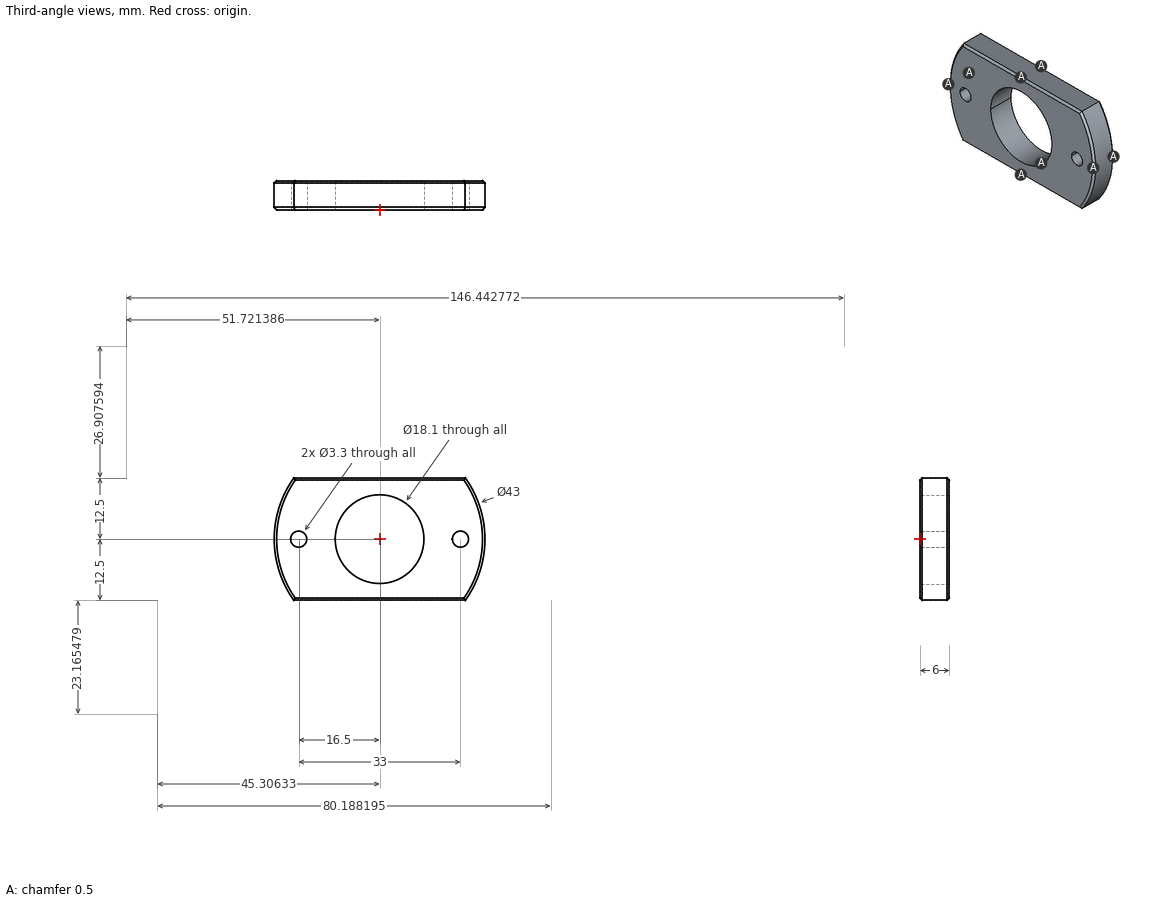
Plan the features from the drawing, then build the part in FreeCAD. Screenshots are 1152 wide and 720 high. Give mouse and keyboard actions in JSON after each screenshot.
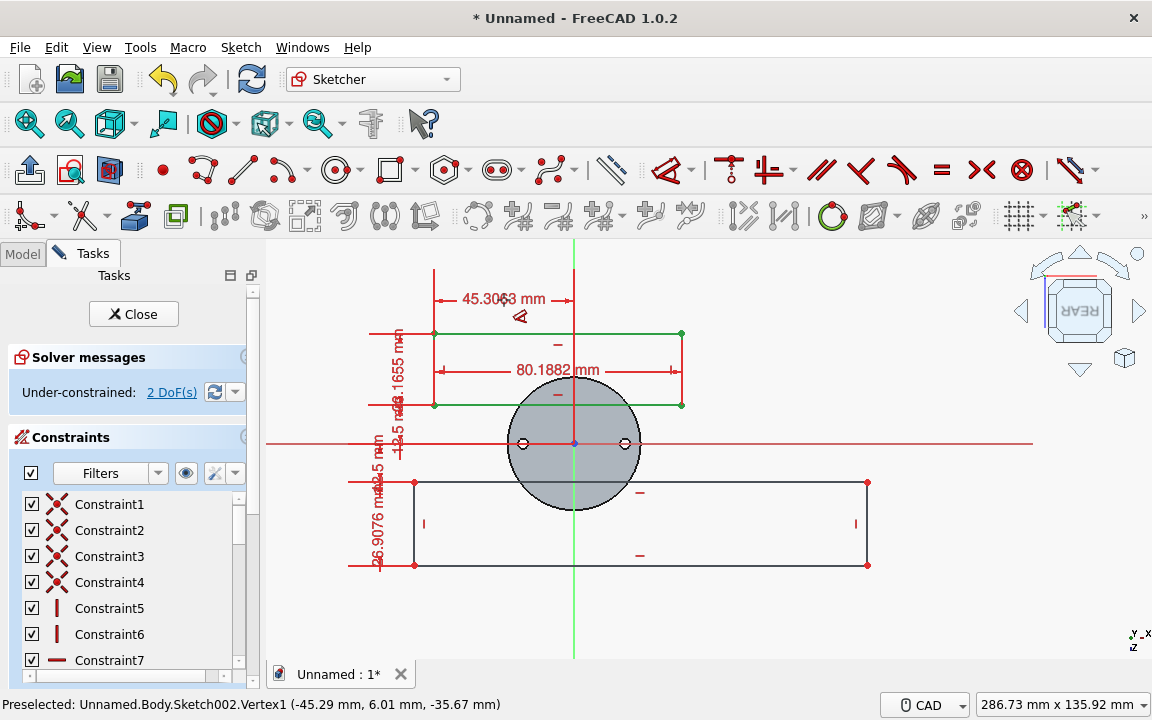
{"action": "left_click", "coordinate": [550, 566]}
{"action": "left_click", "coordinate": [641, 600]}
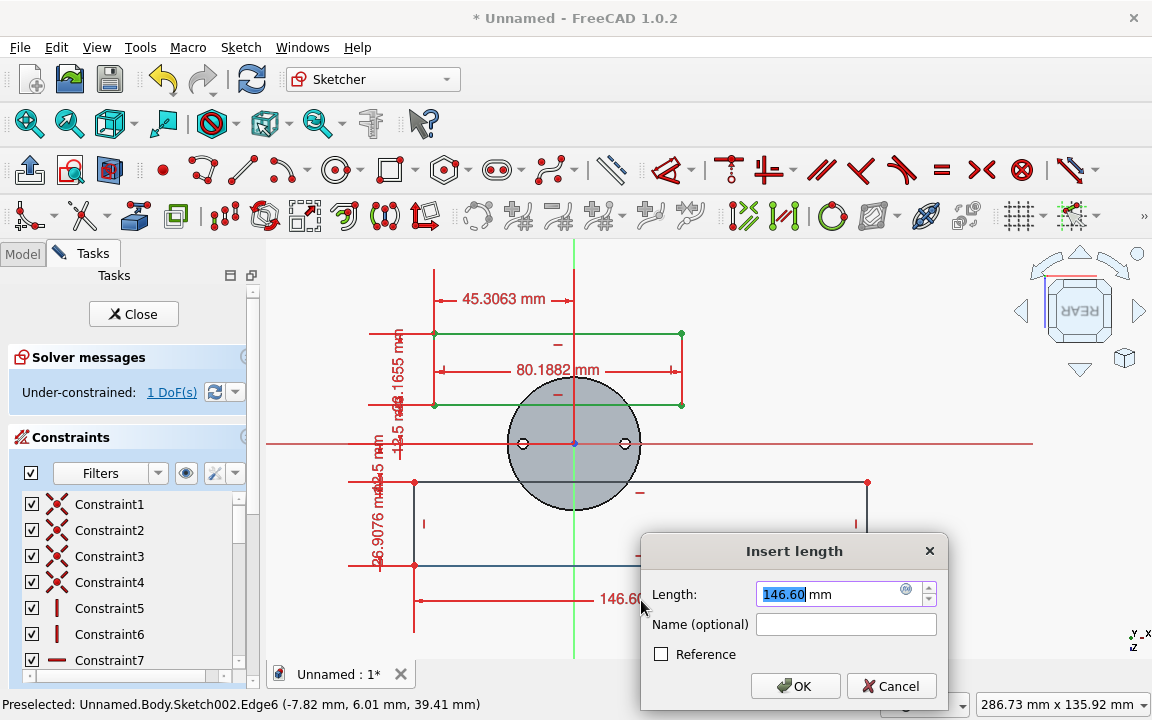
{"action": "type", "text": "146.442772"}
{"action": "key", "text": "Return"}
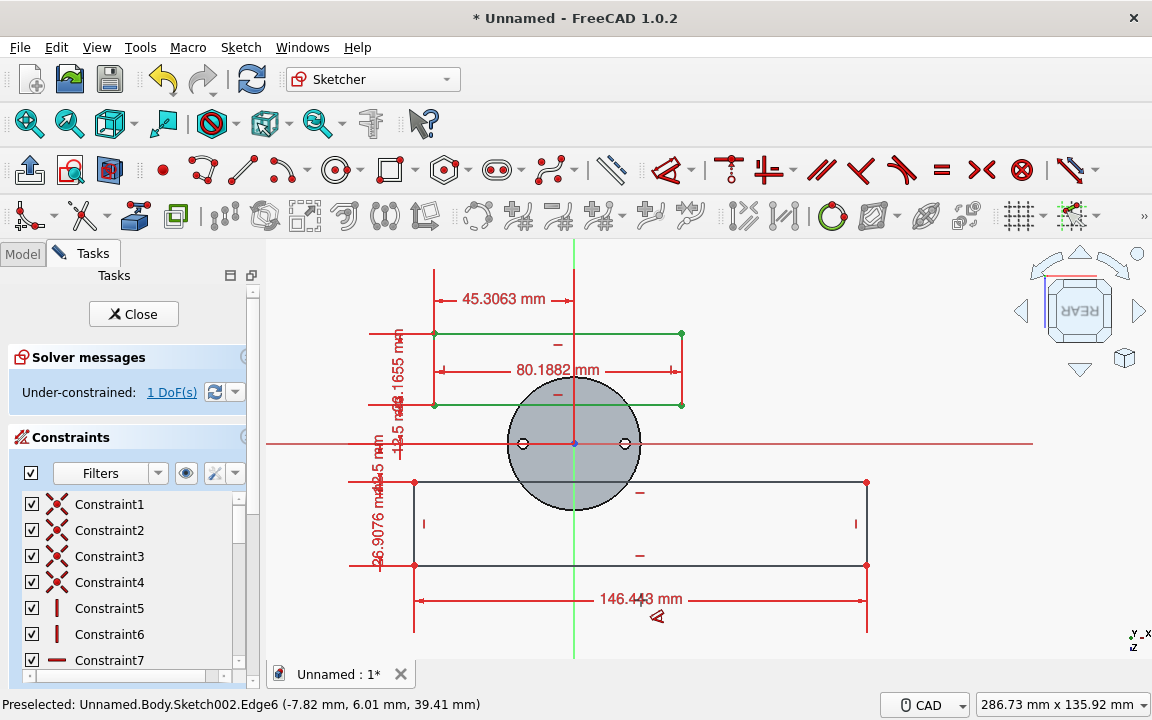
{"action": "left_click", "coordinate": [414, 482]}
{"action": "left_click", "coordinate": [494, 516]}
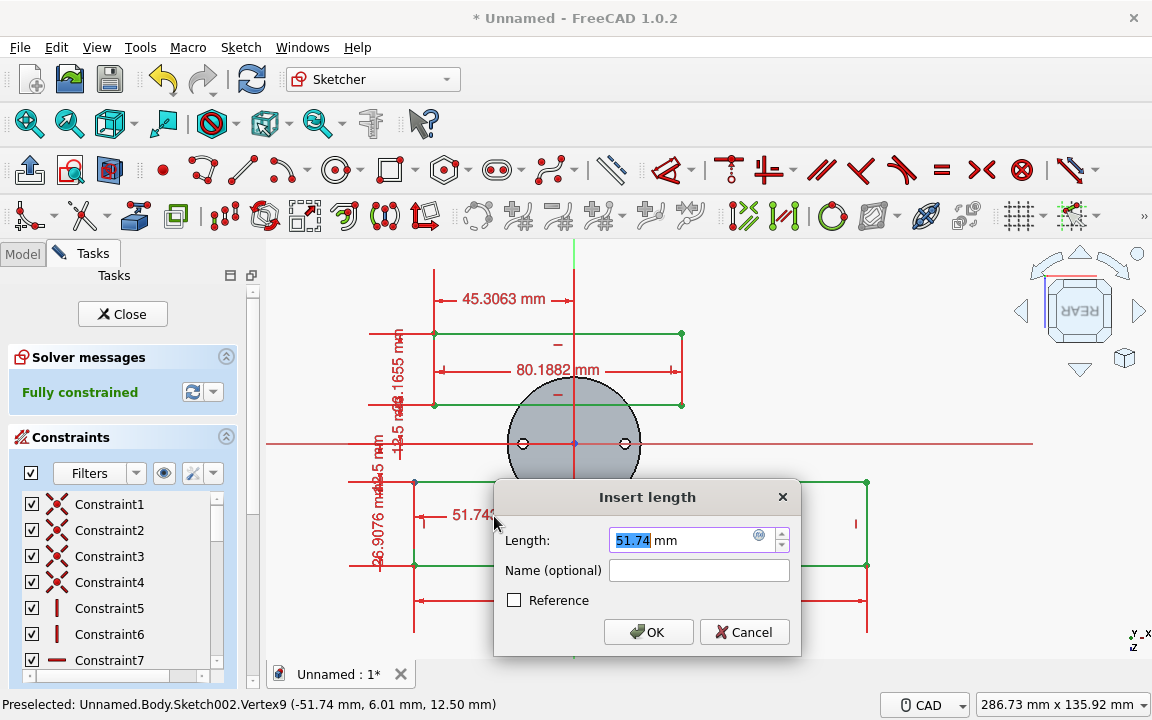
{"action": "type", "text": "51.721386"}
{"action": "key", "text": "Return"}
{"action": "key", "text": "Escape"}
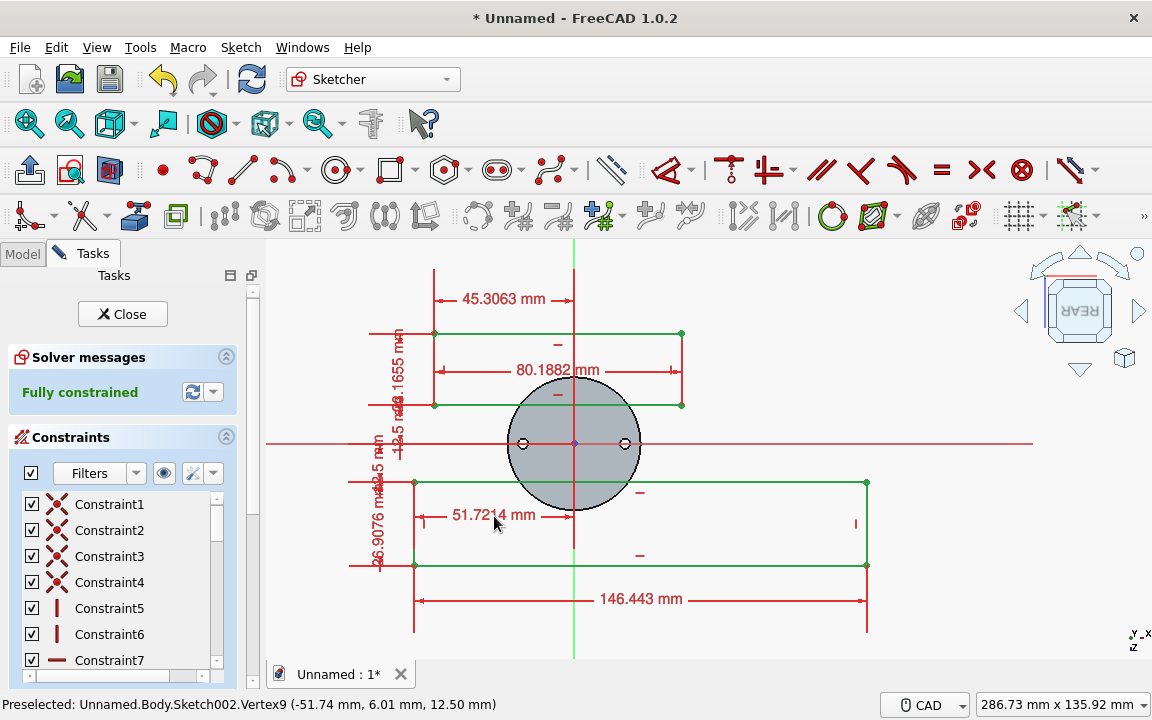
{"action": "left_click", "coordinate": [123, 314]}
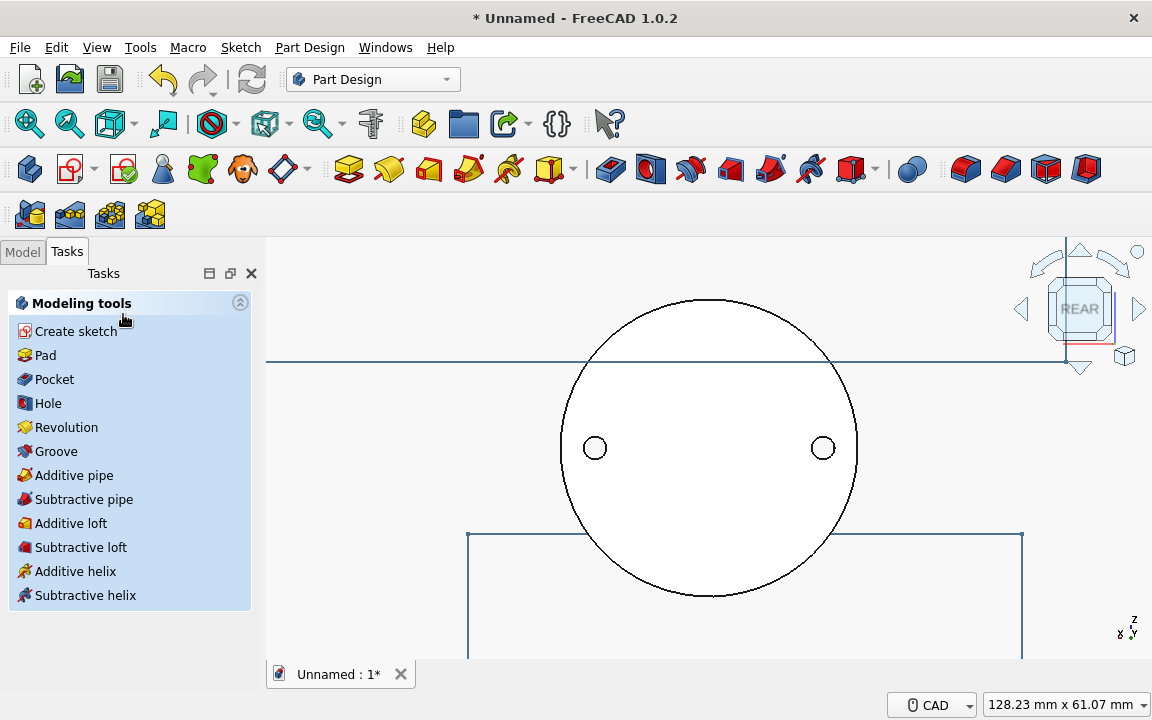
{"action": "left_click", "coordinate": [612, 170]}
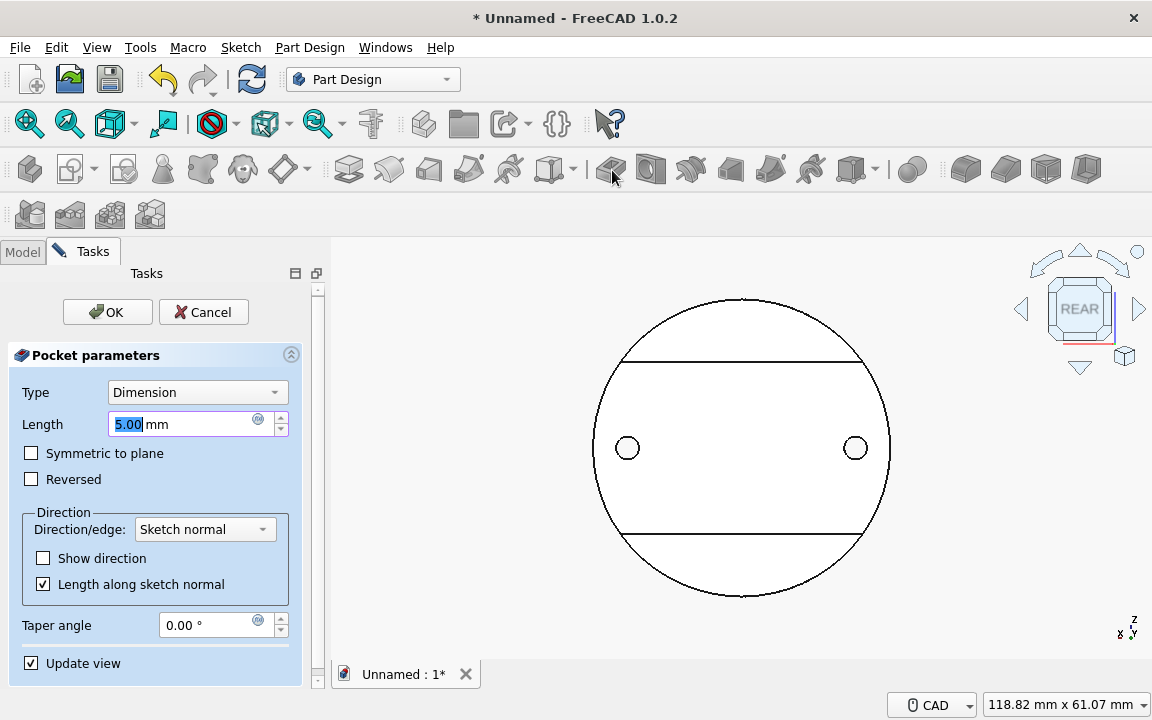
{"action": "left_click", "coordinate": [198, 392]}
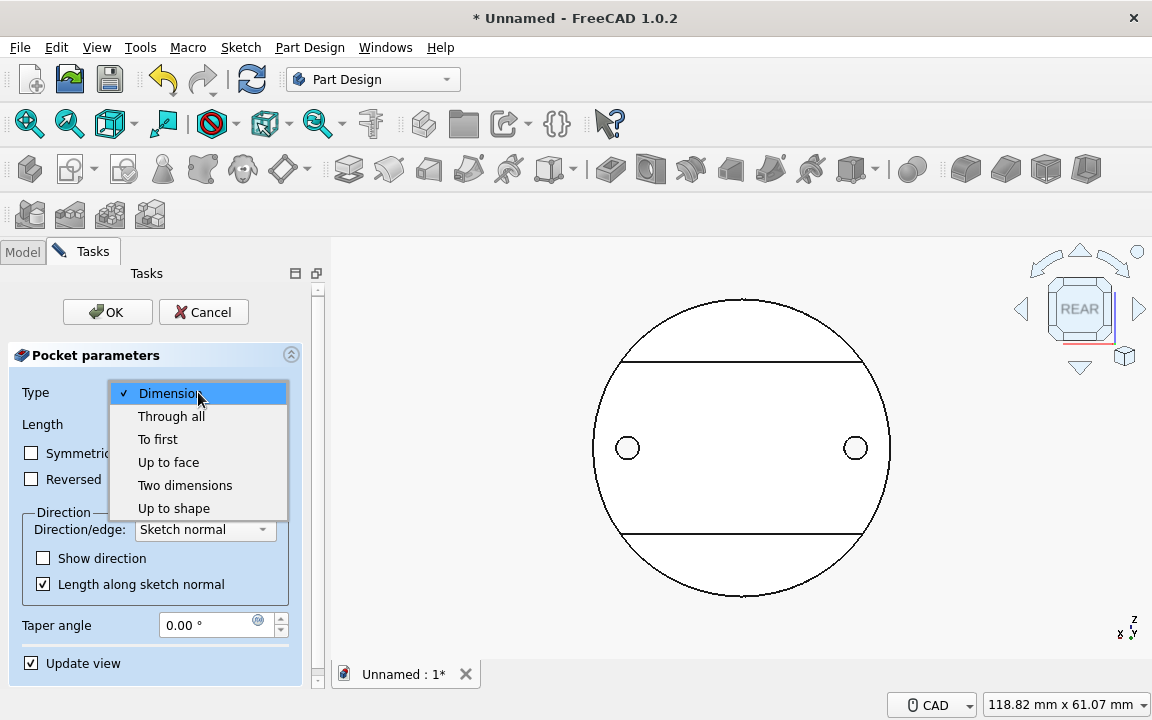
{"action": "left_click", "coordinate": [198, 416]}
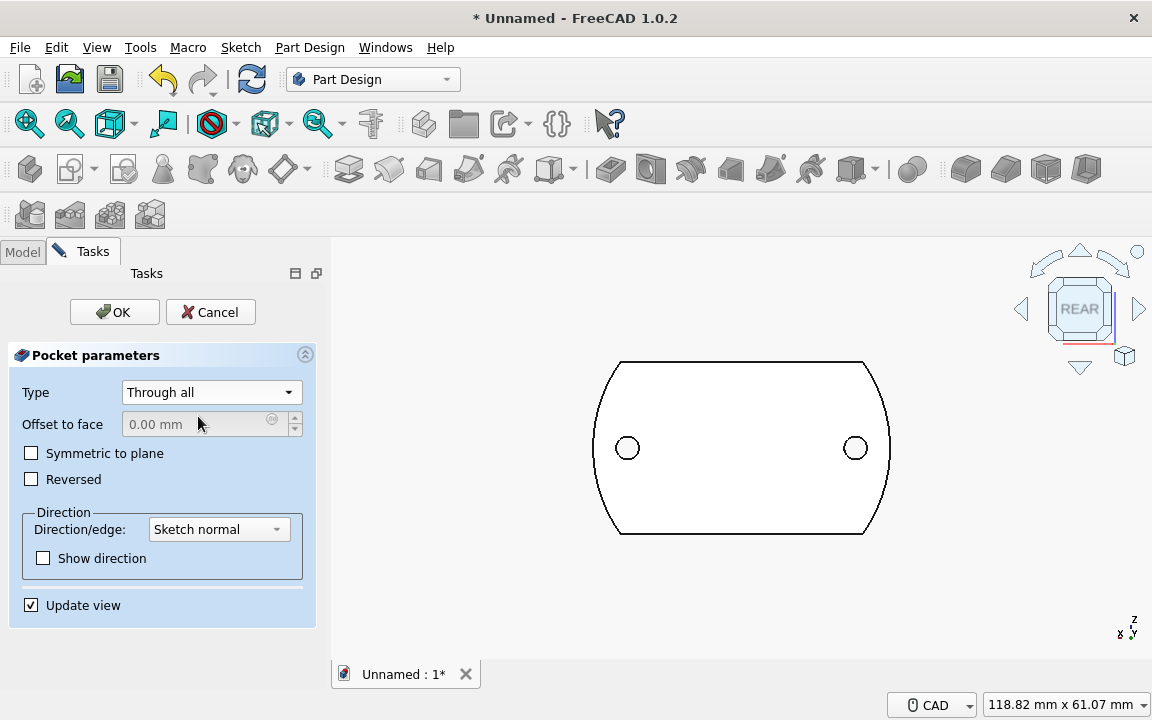
{"action": "left_click", "coordinate": [115, 312]}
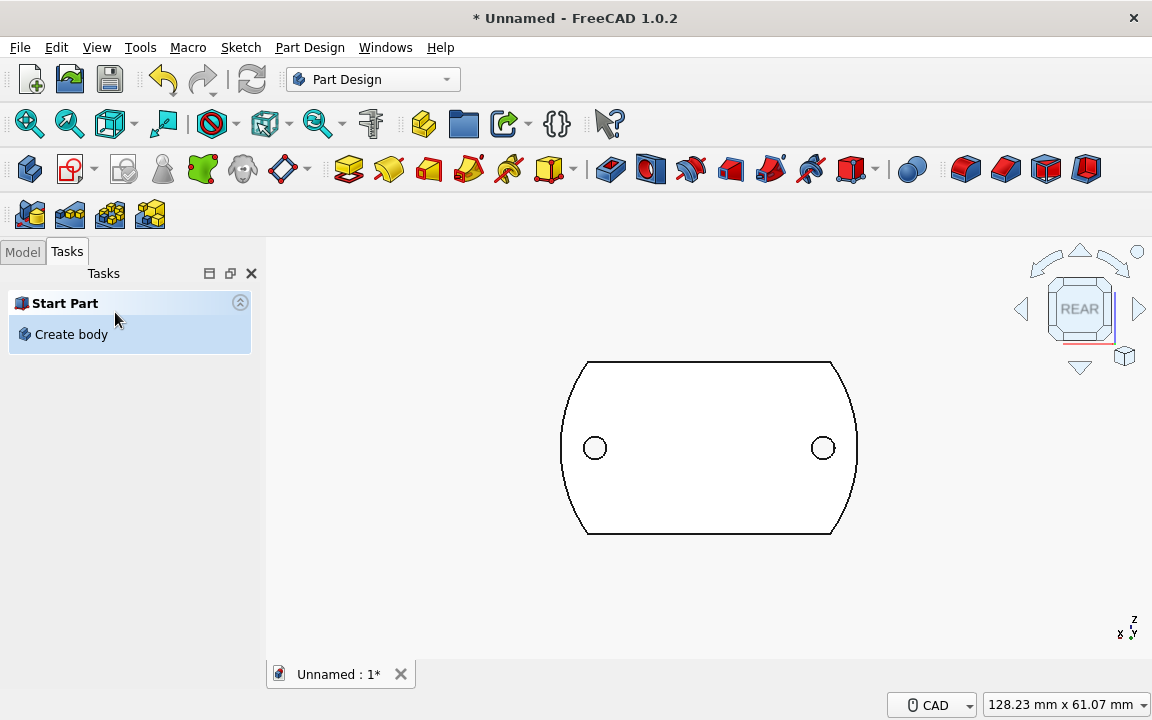
{"action": "left_click", "coordinate": [30, 124]}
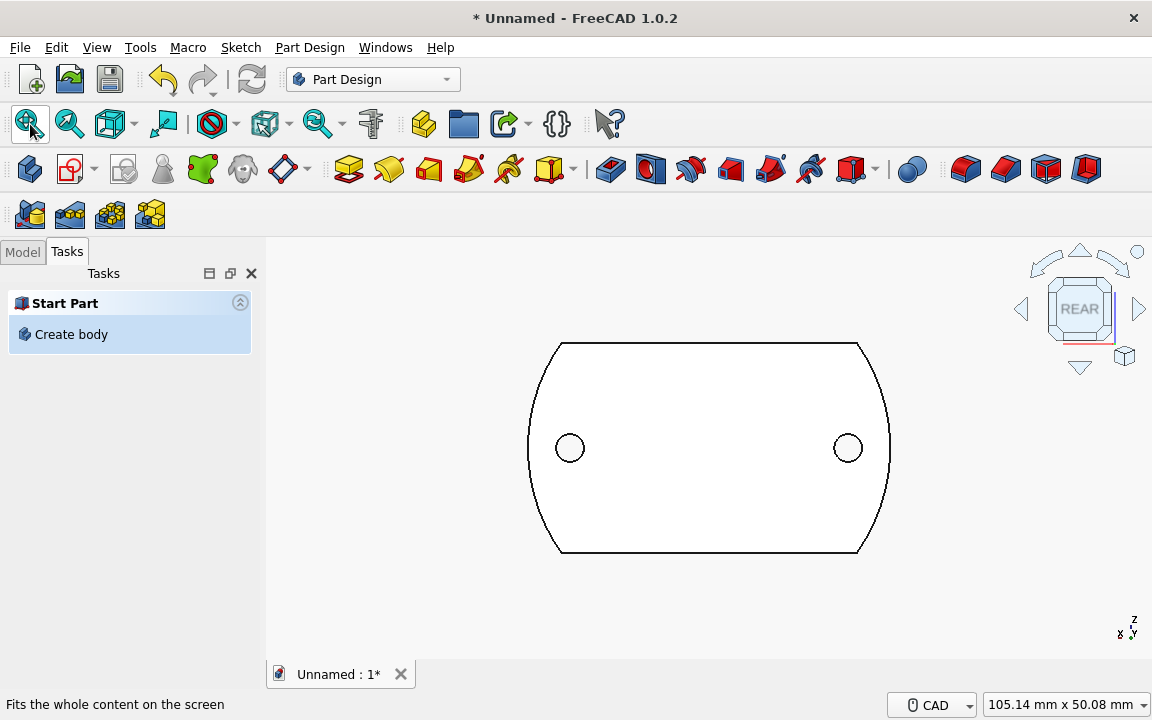
{"action": "left_click", "coordinate": [709, 447]}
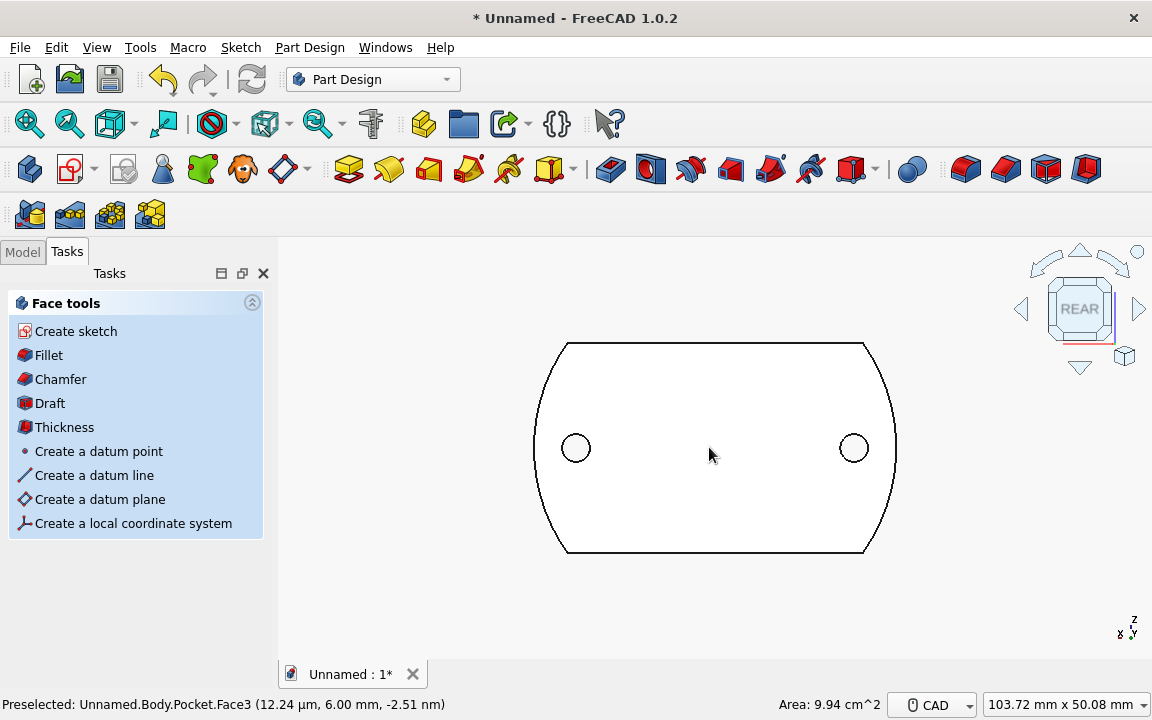
{"action": "left_click", "coordinate": [70, 170]}